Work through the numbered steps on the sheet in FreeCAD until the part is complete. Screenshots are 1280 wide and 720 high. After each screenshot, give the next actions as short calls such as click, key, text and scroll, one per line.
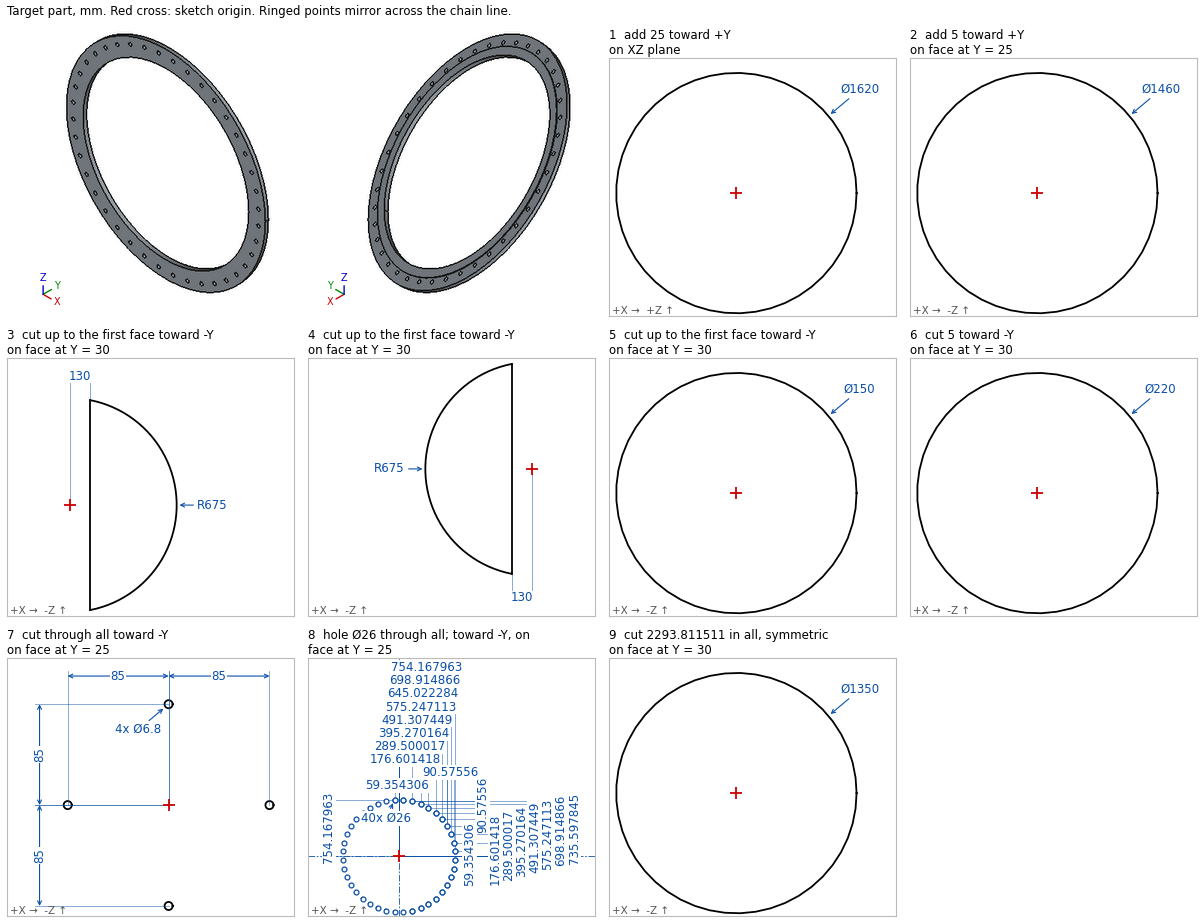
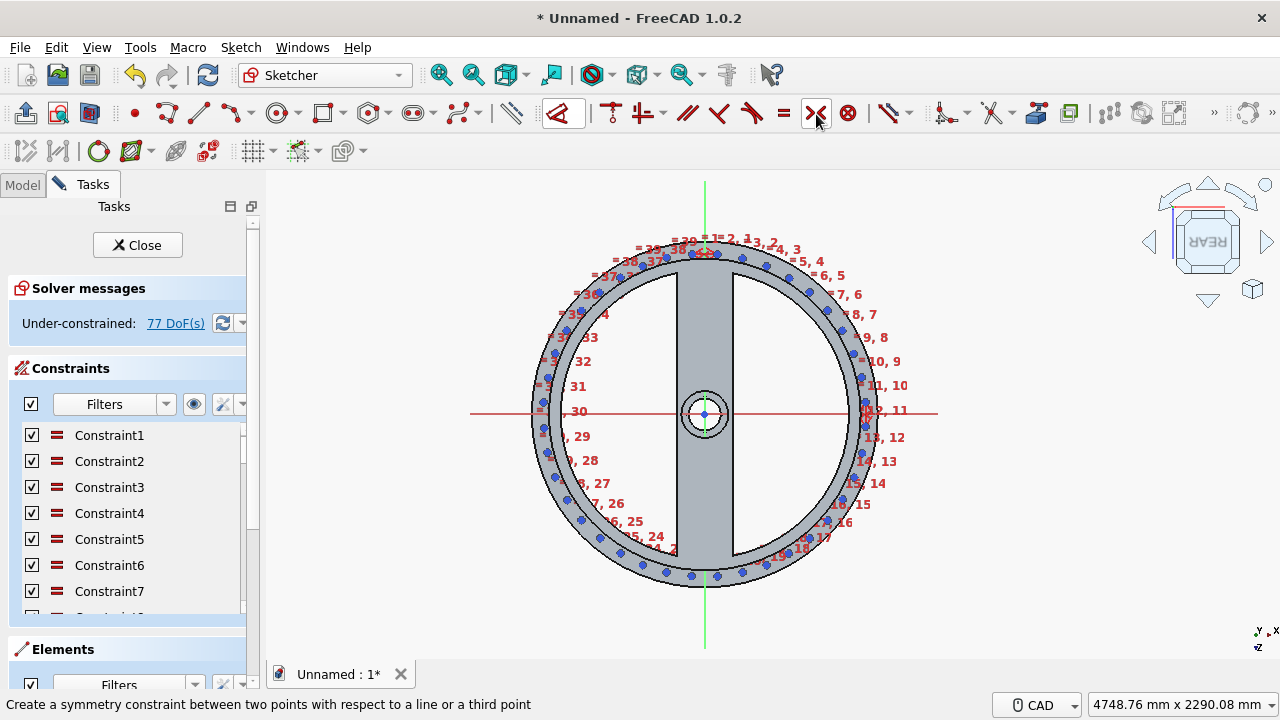
click(862, 377)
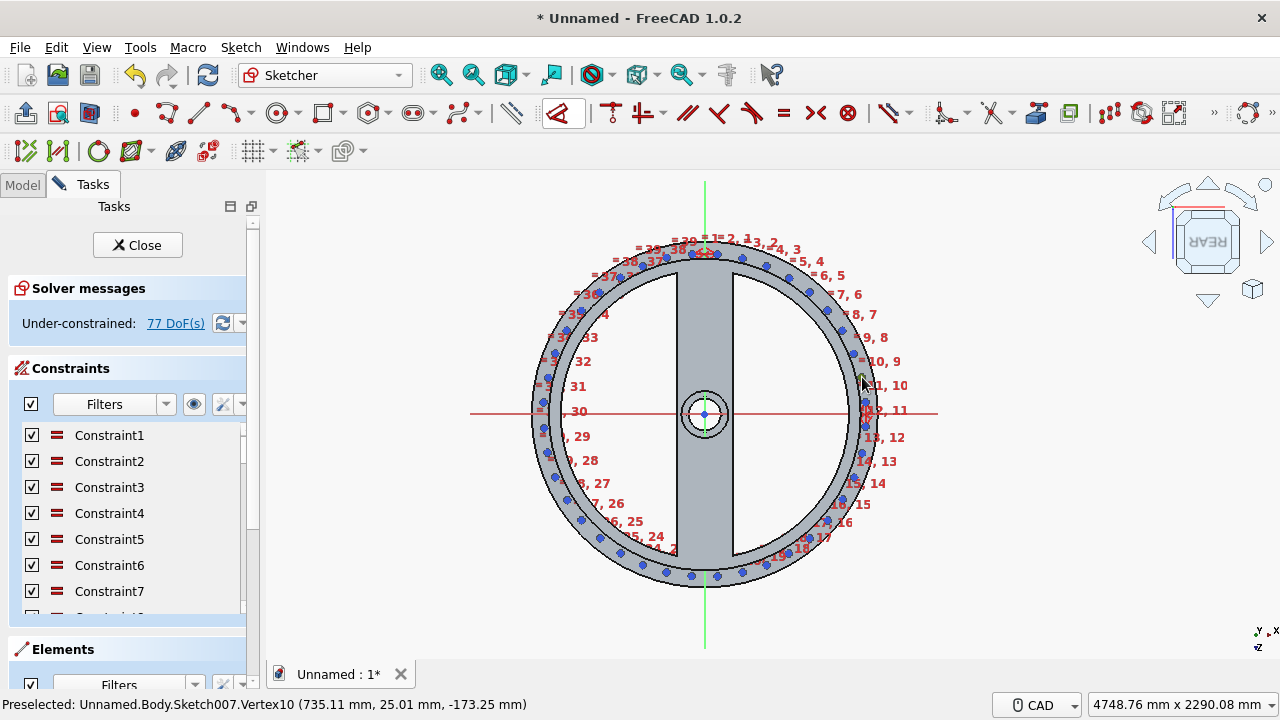
click(862, 453)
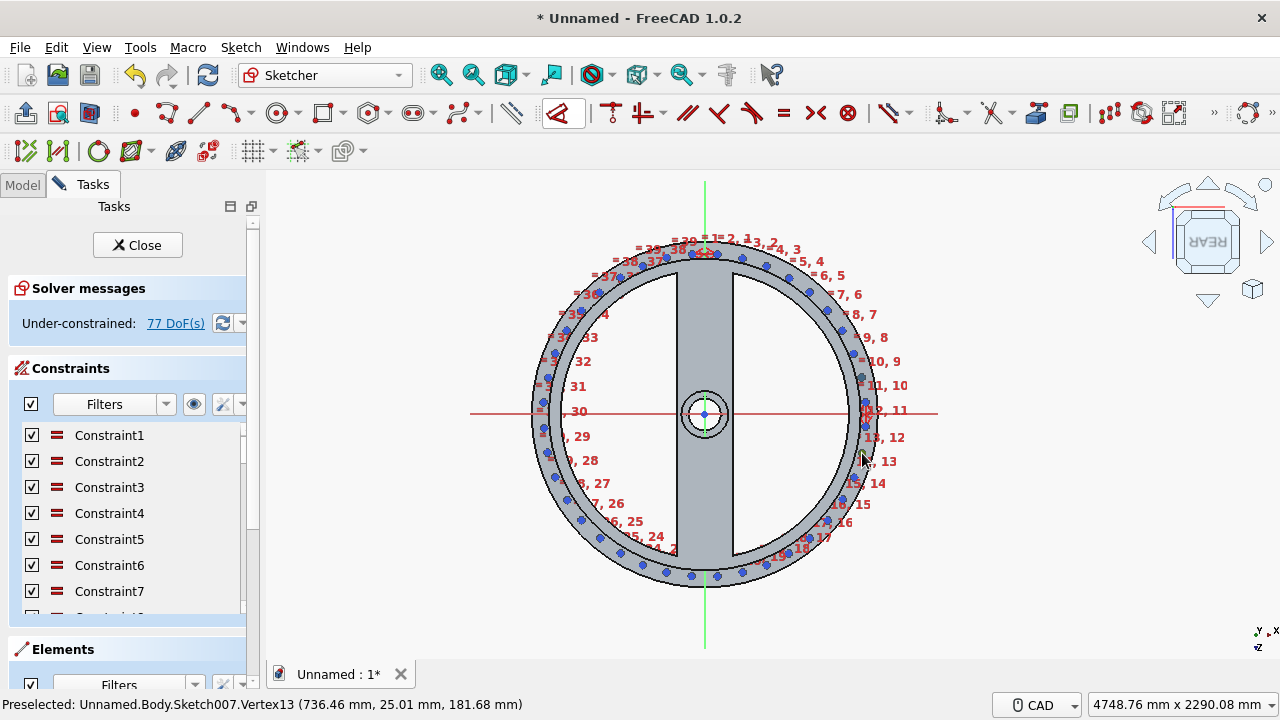
click(470, 414)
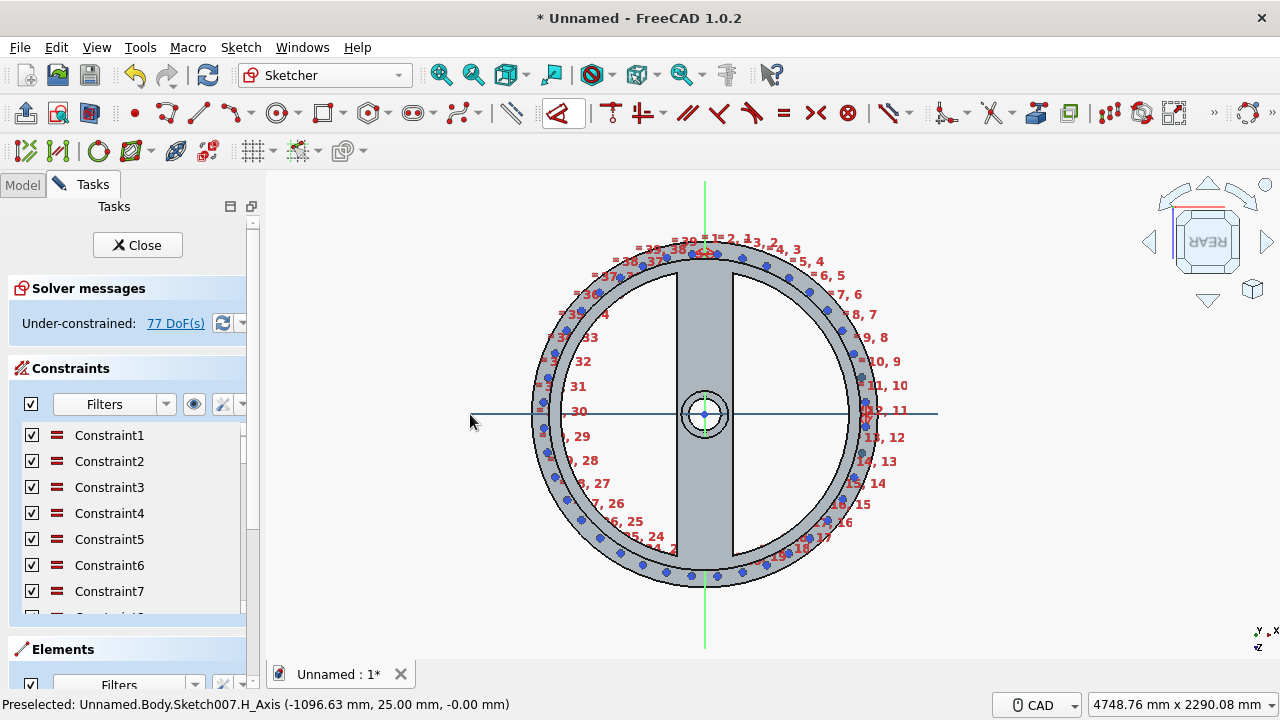
click(816, 114)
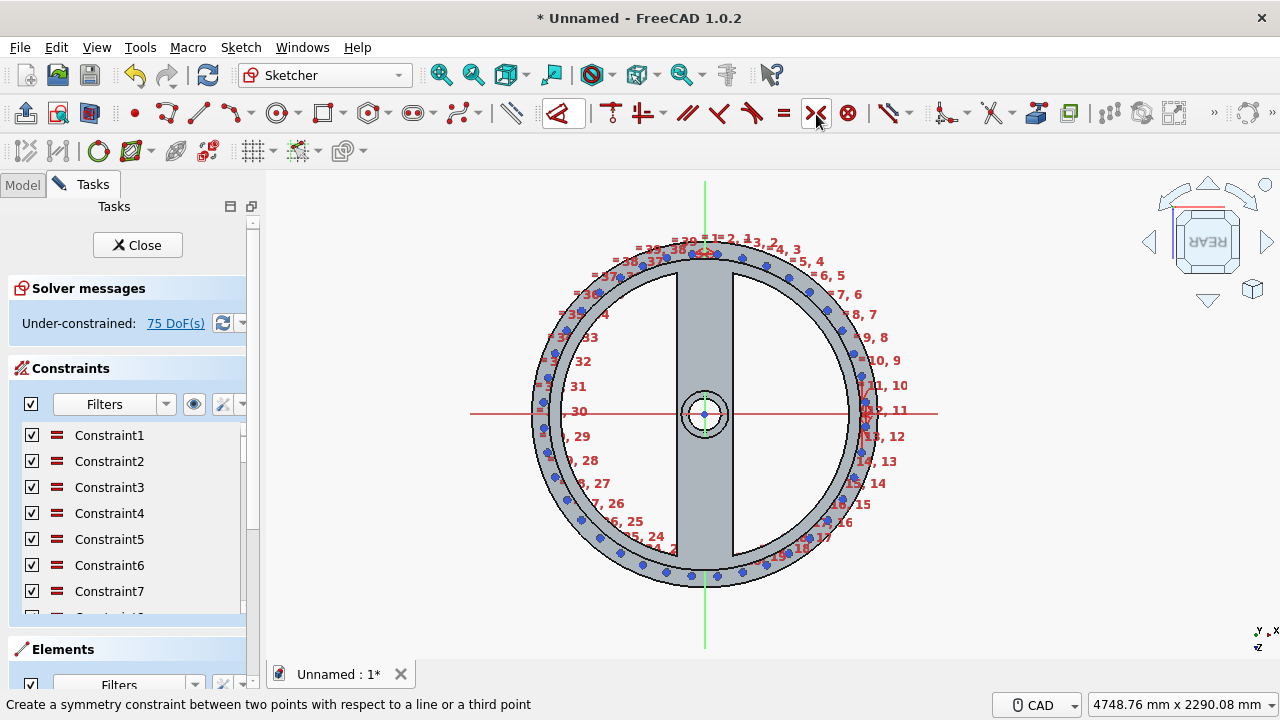
click(854, 354)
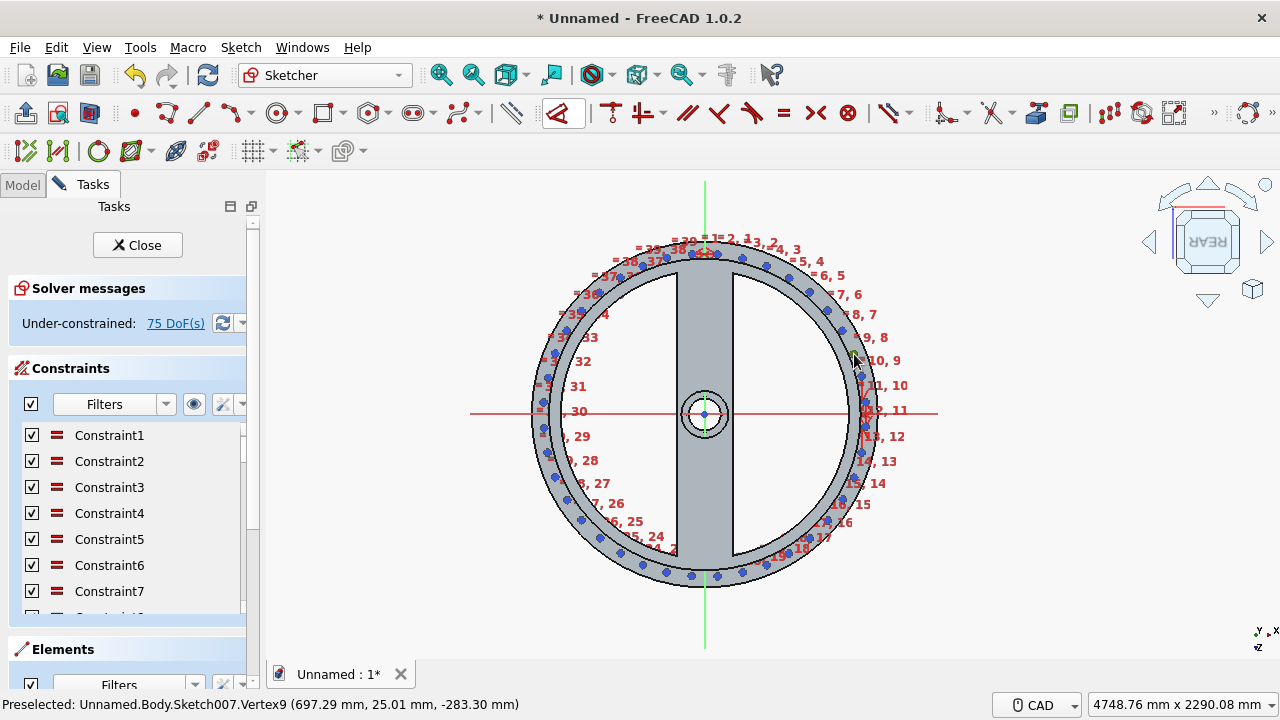
click(854, 478)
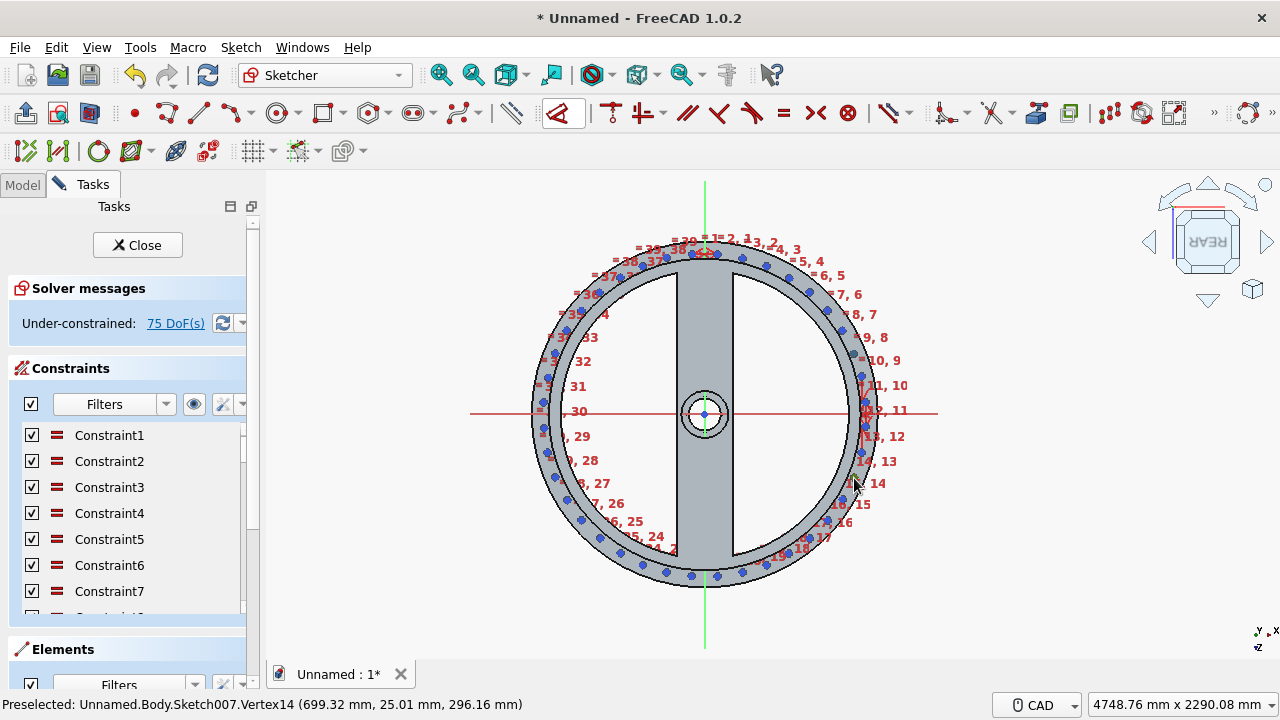
click(470, 414)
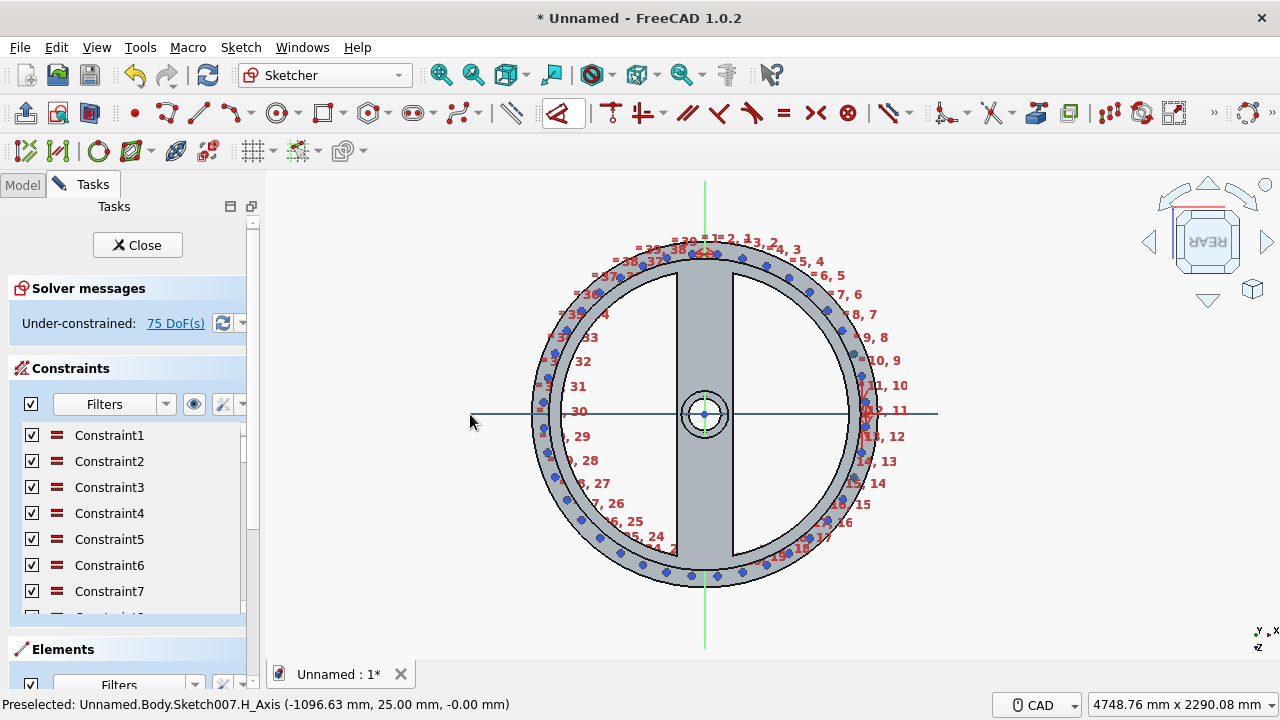
click(816, 114)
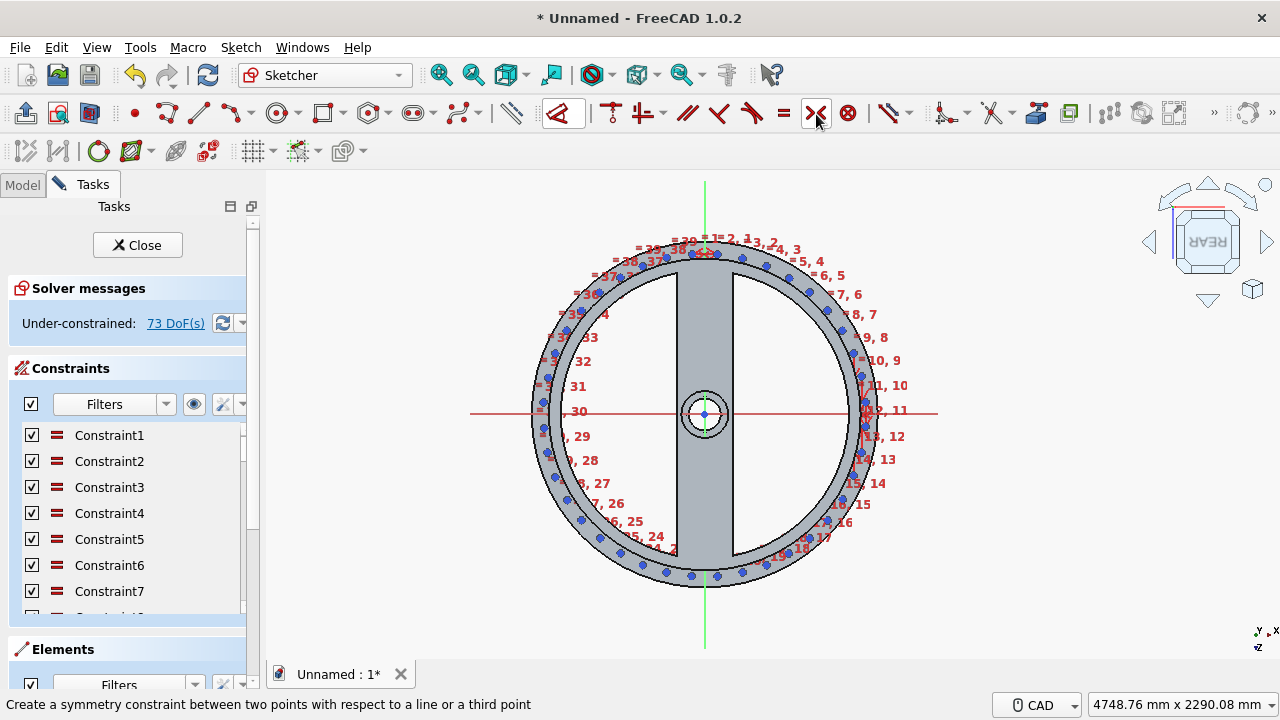
click(842, 331)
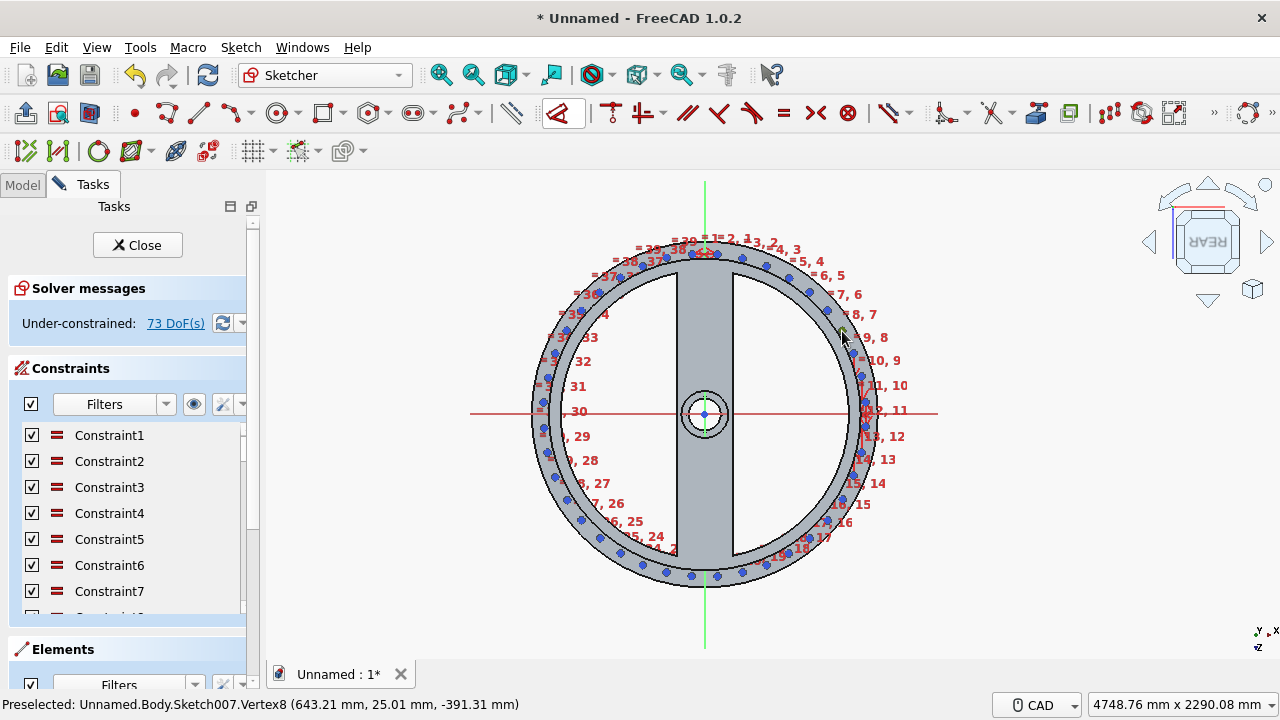
click(843, 500)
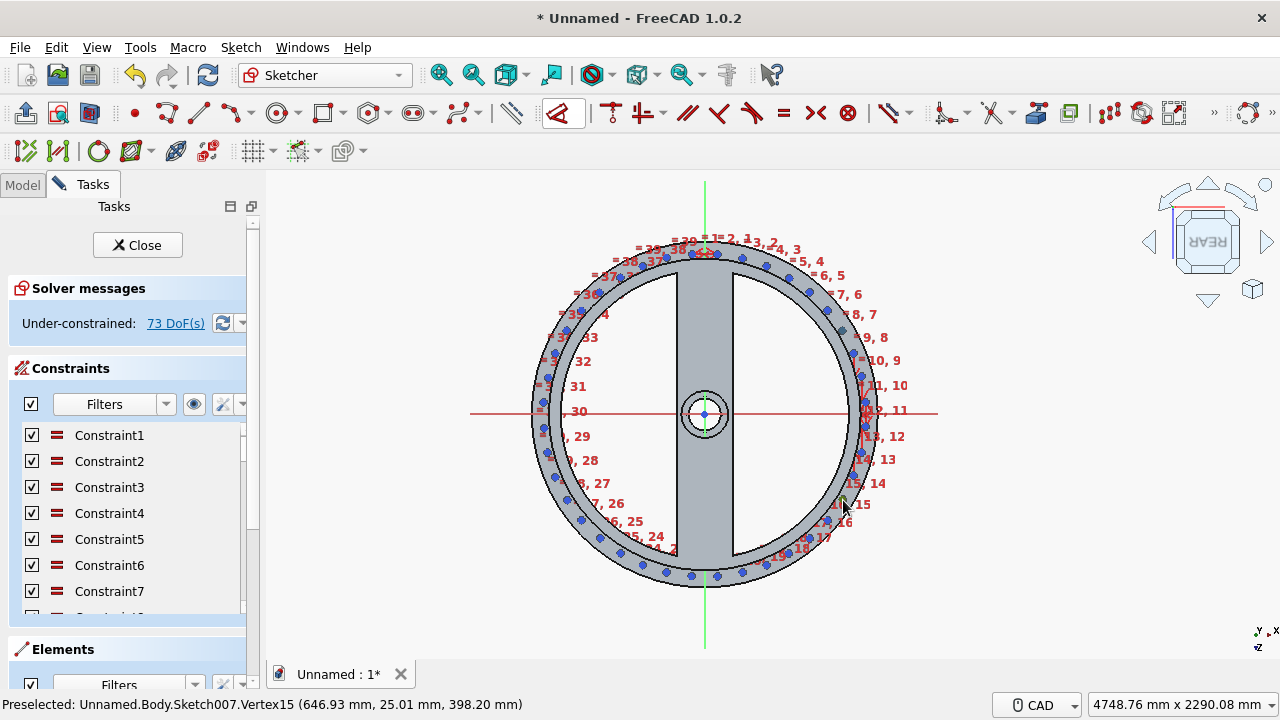
click(470, 414)